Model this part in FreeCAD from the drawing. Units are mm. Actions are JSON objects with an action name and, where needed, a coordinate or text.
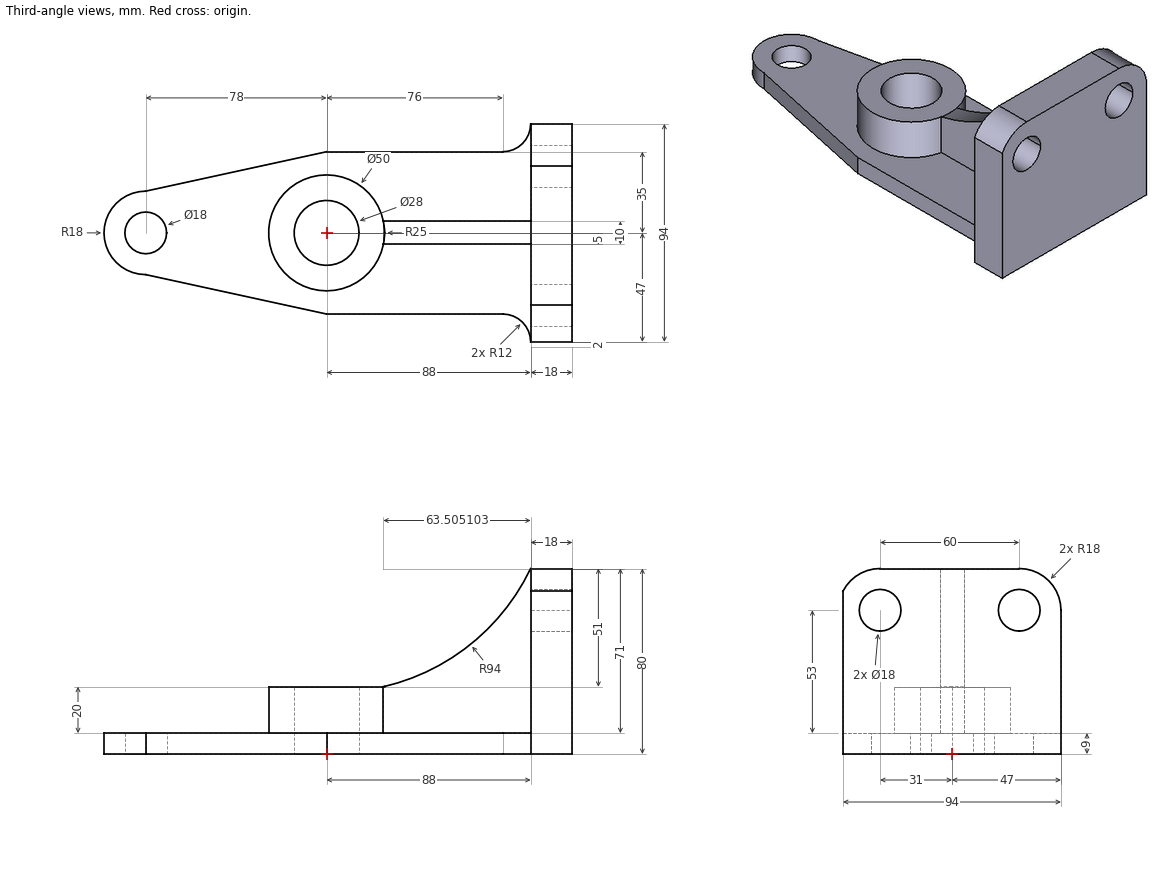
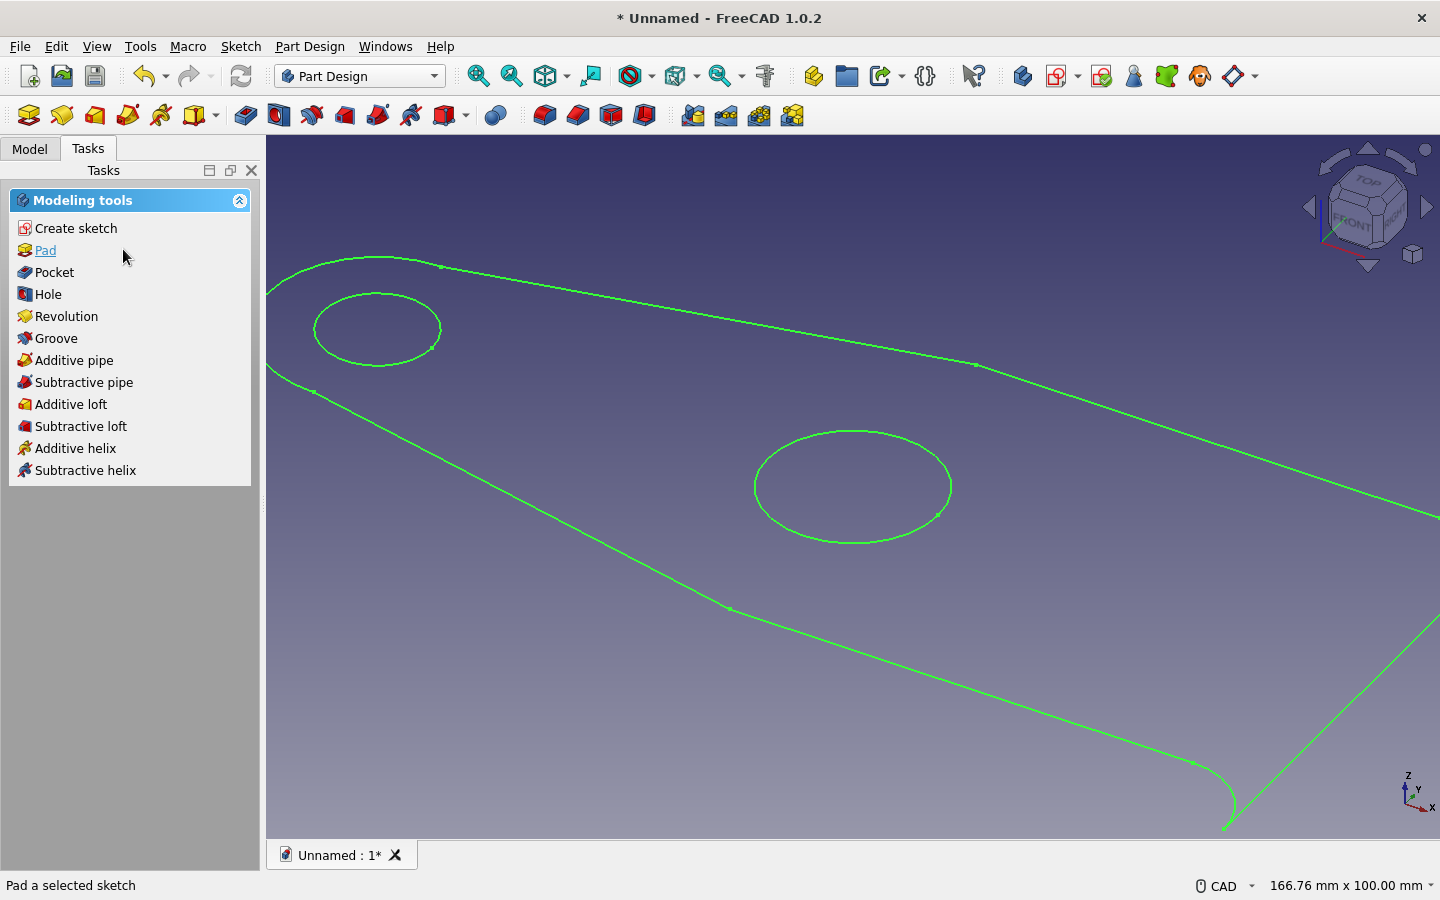
{"action": "left_click", "coordinate": [29, 116]}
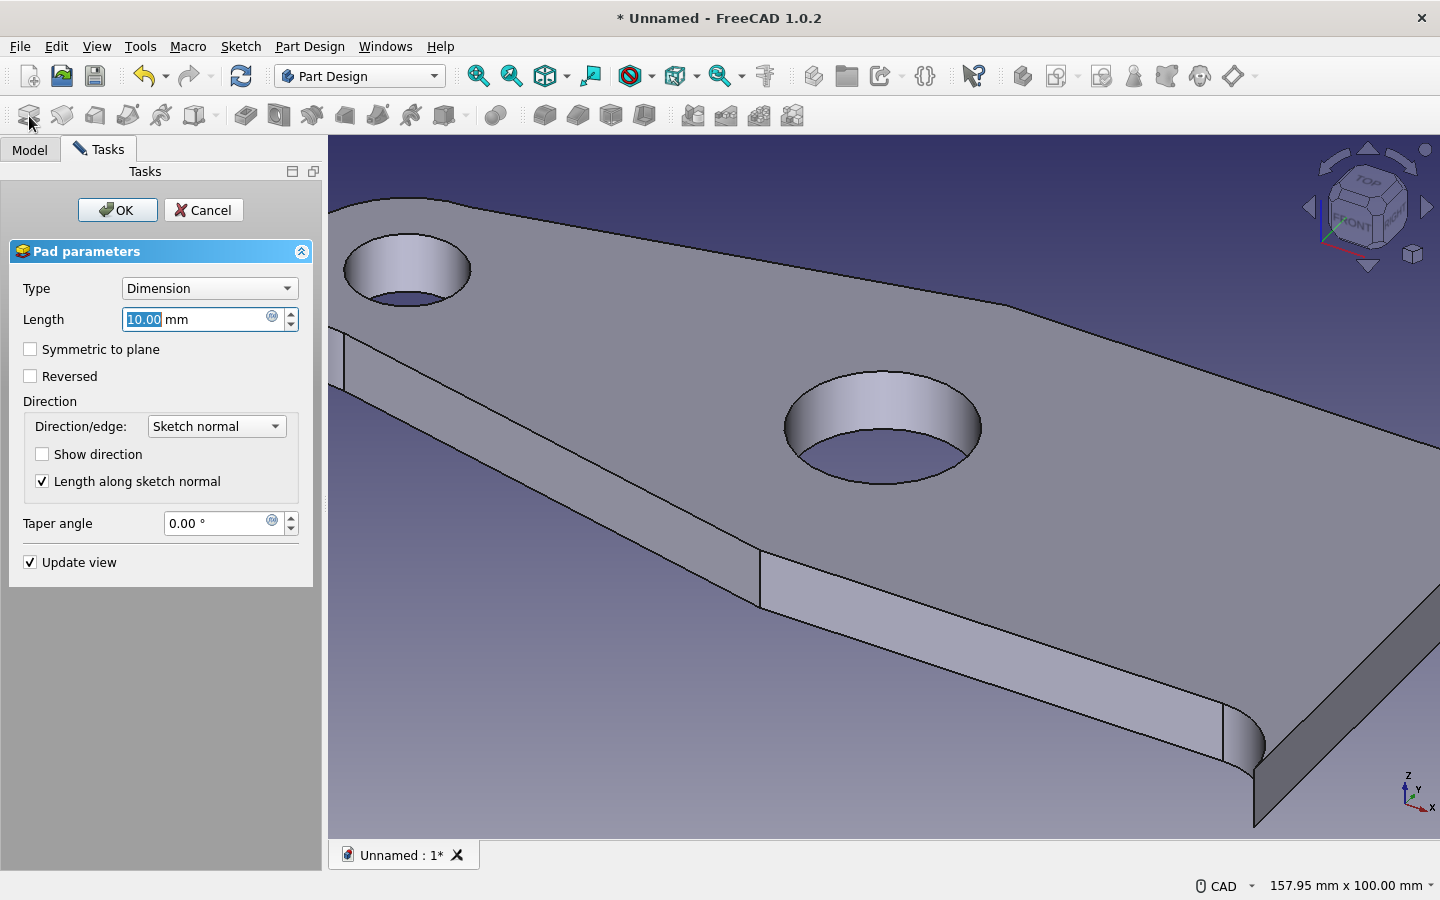
{"action": "type", "text": "9"}
{"action": "key", "text": "Tab"}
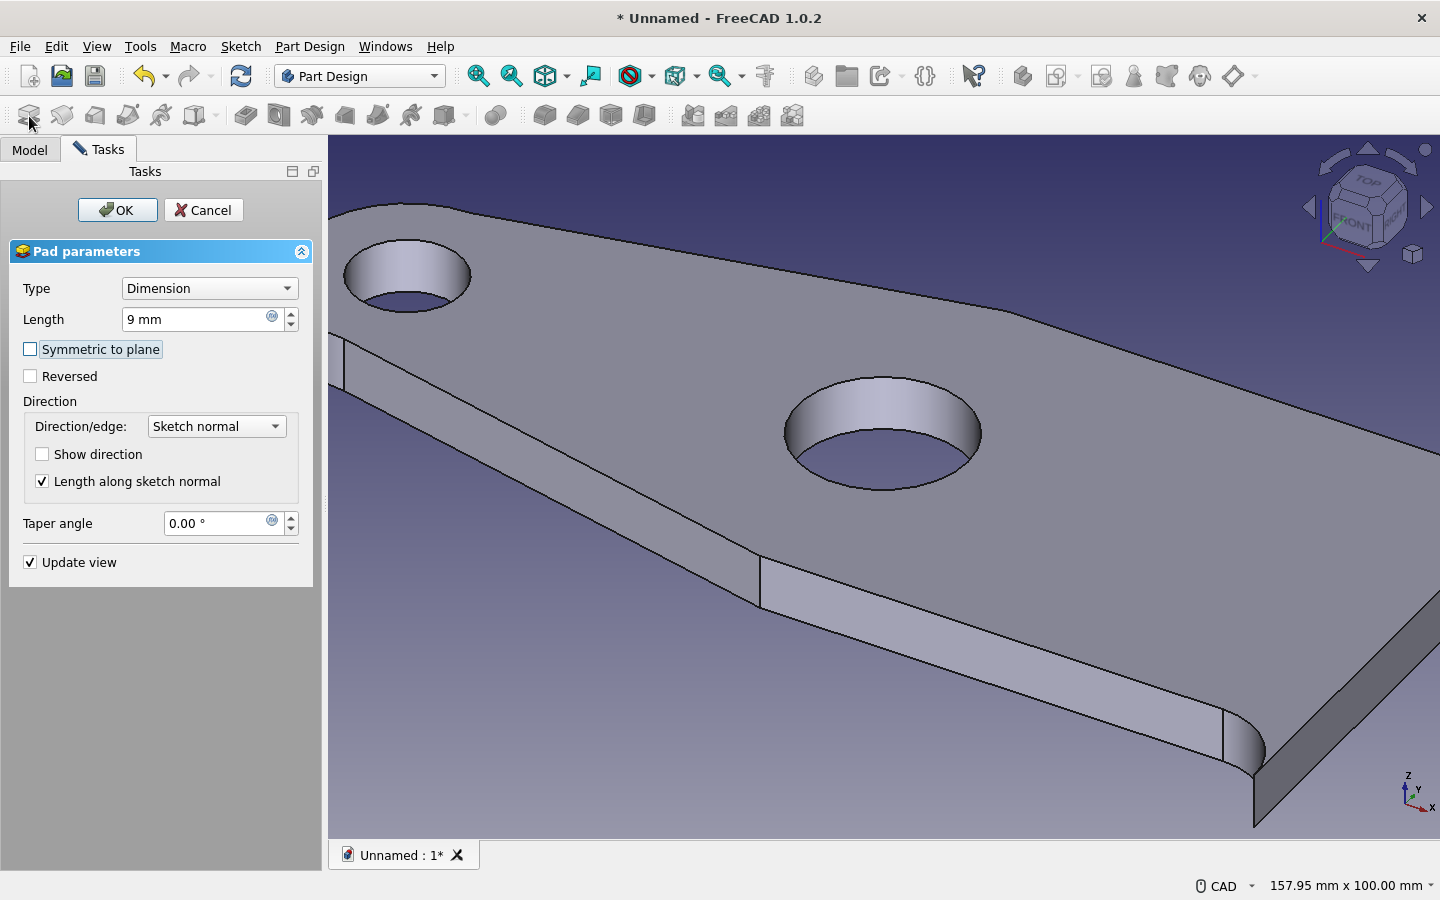
{"action": "left_click", "coordinate": [118, 210]}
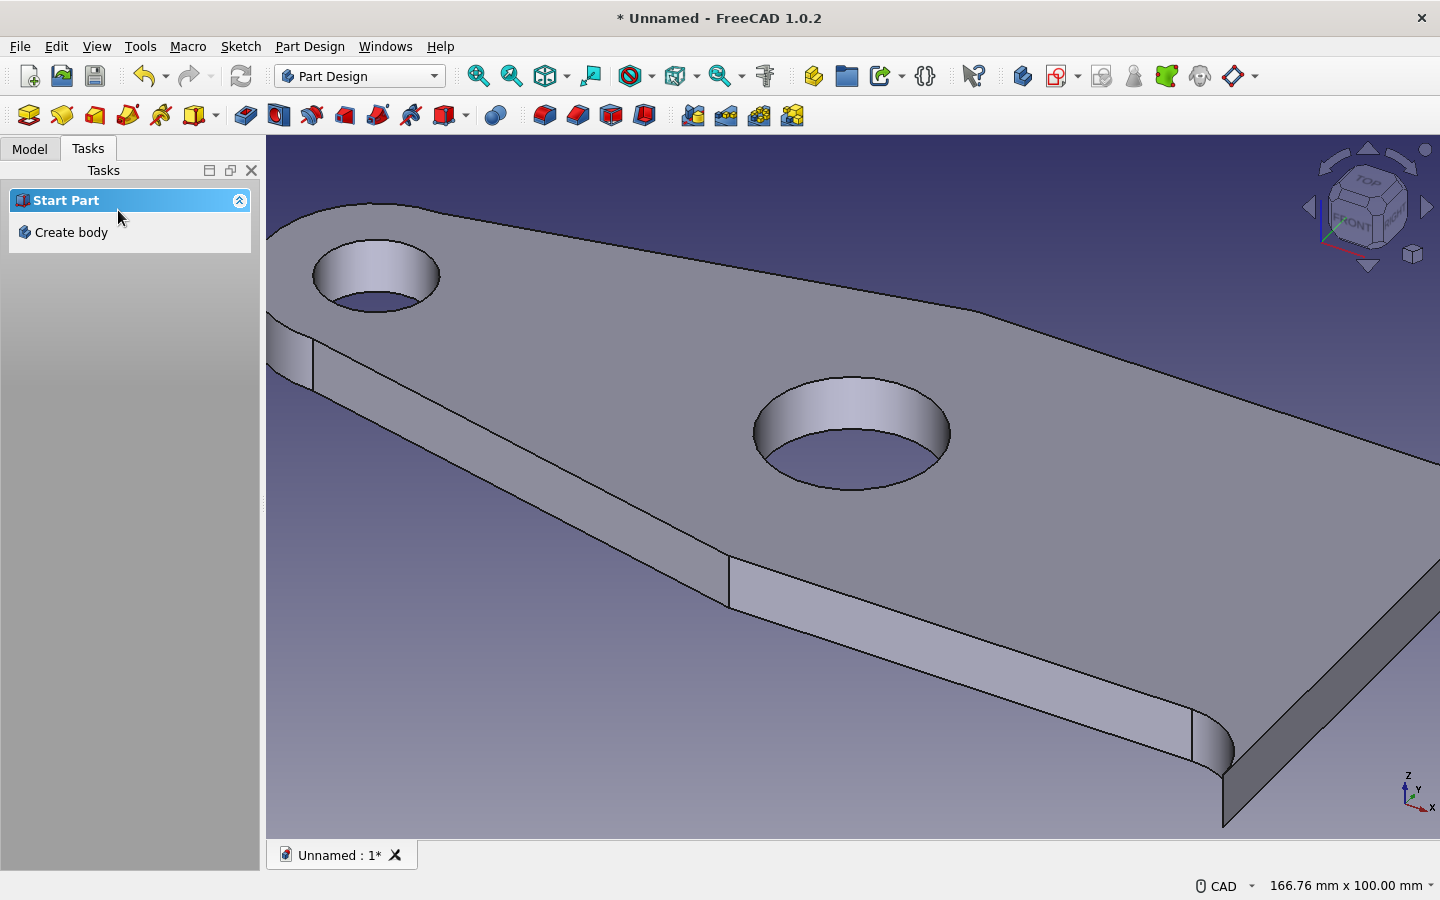
{"action": "key", "text": "v f"}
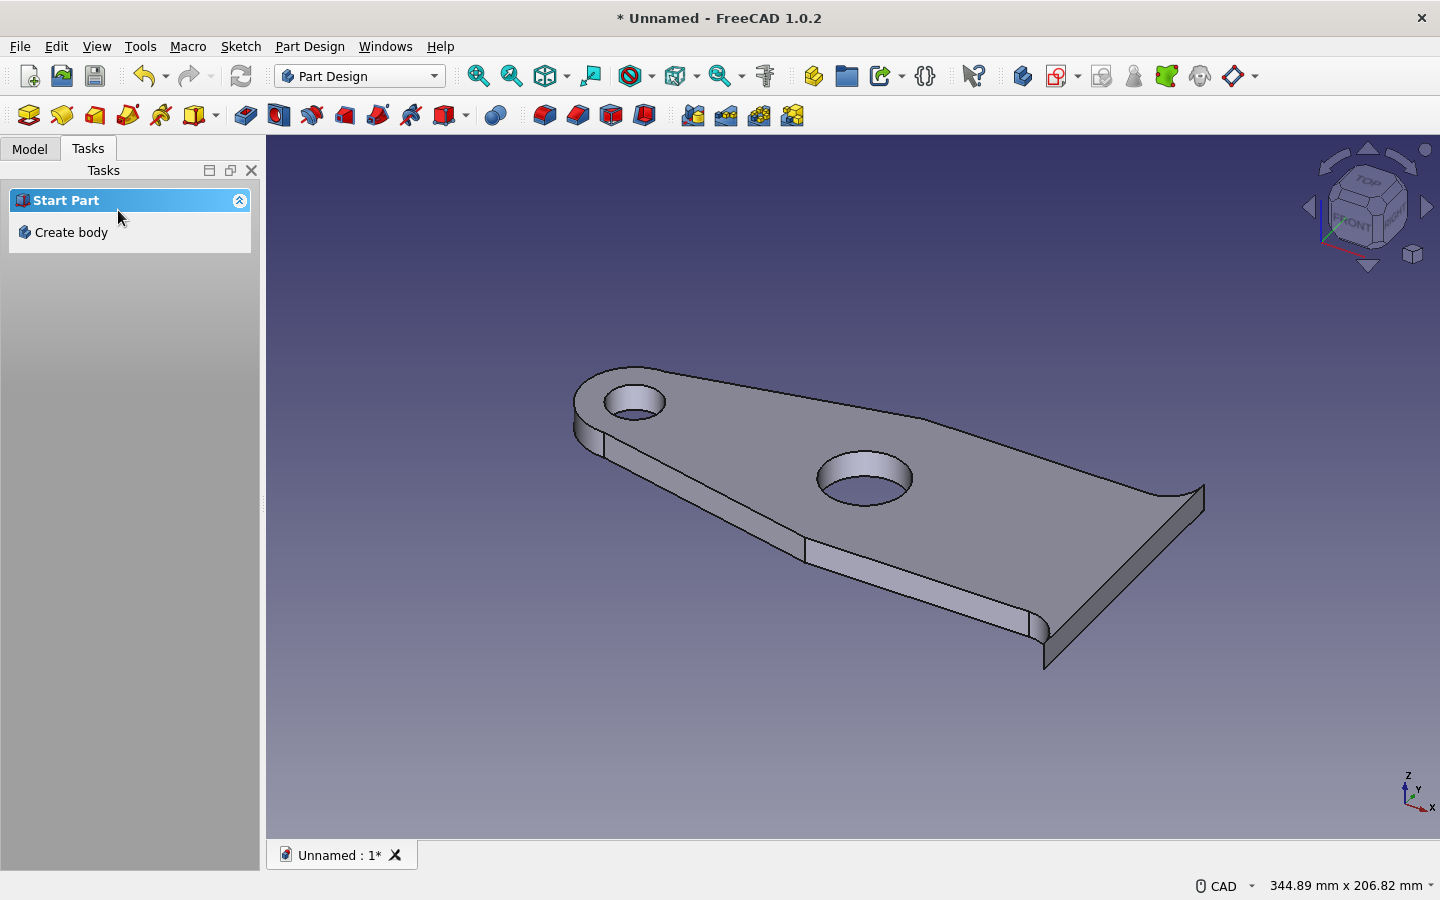
{"action": "left_click", "coordinate": [1023, 76]}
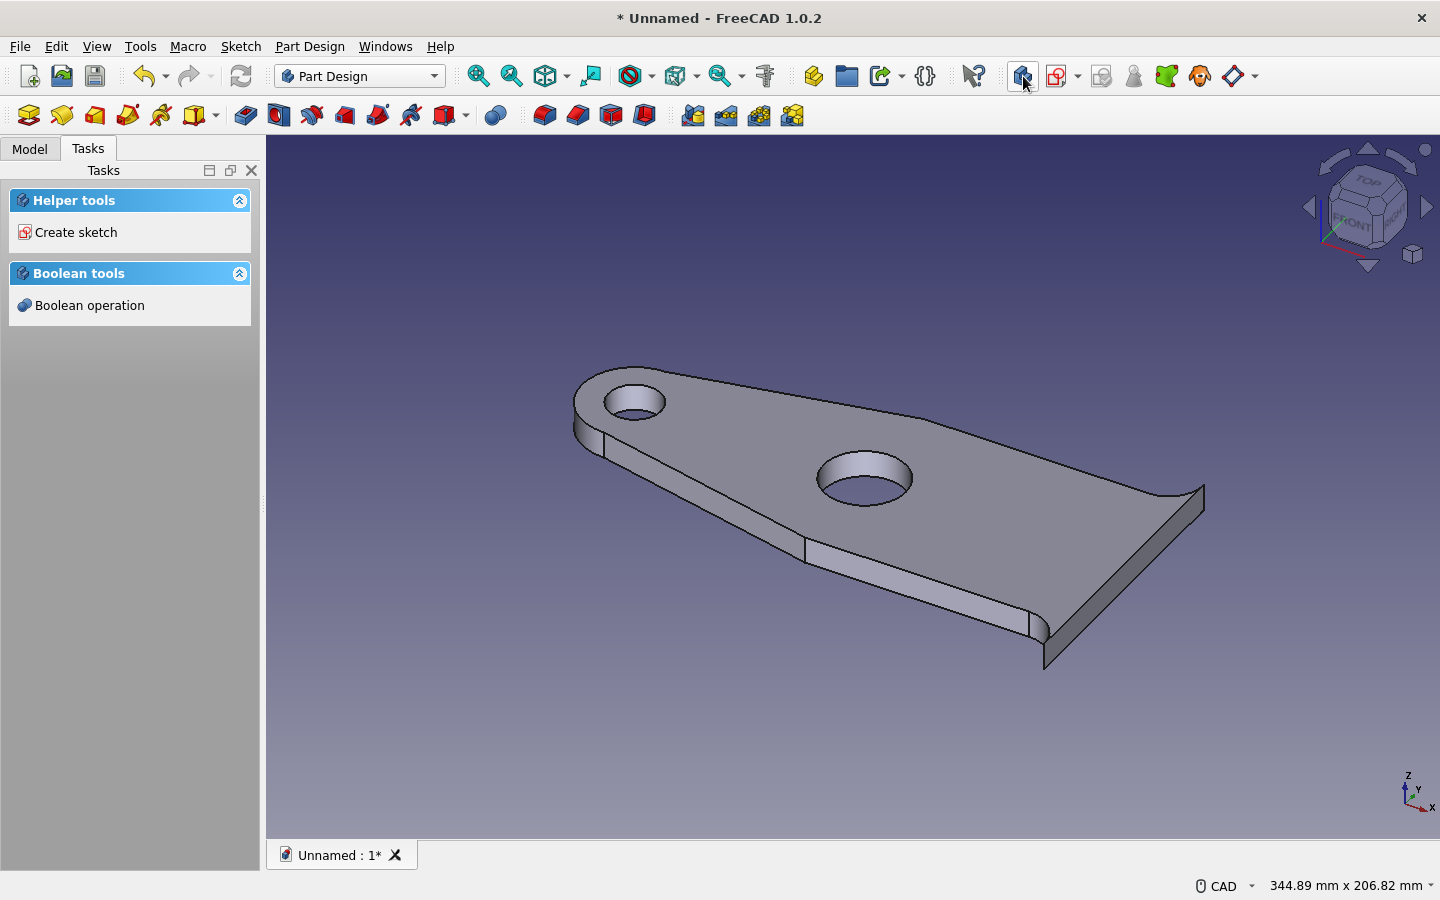
{"action": "left_click", "coordinate": [30, 148]}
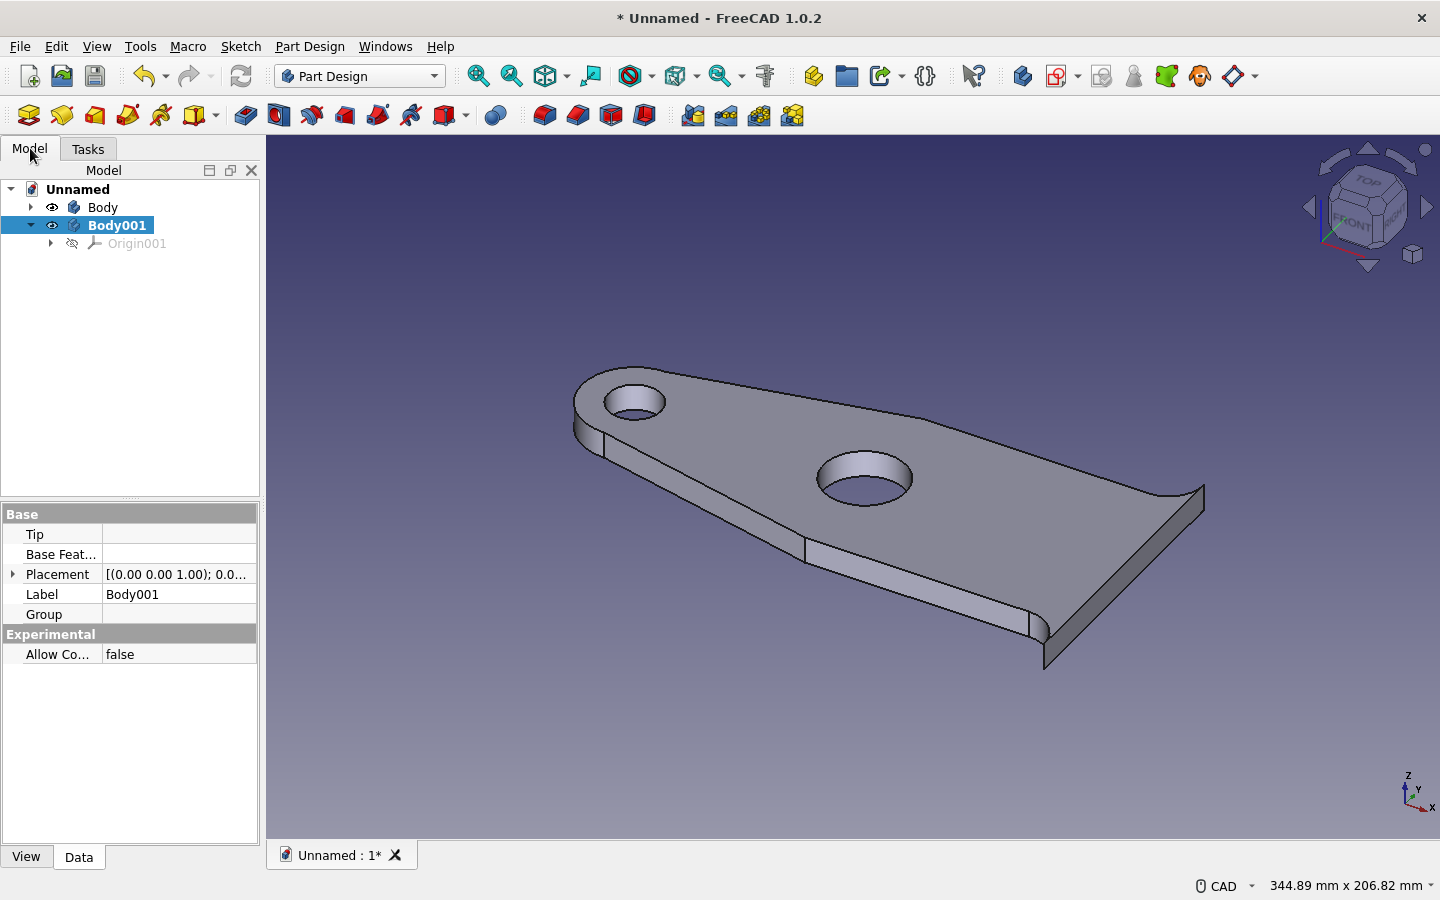
{"action": "left_click", "coordinate": [51, 243]}